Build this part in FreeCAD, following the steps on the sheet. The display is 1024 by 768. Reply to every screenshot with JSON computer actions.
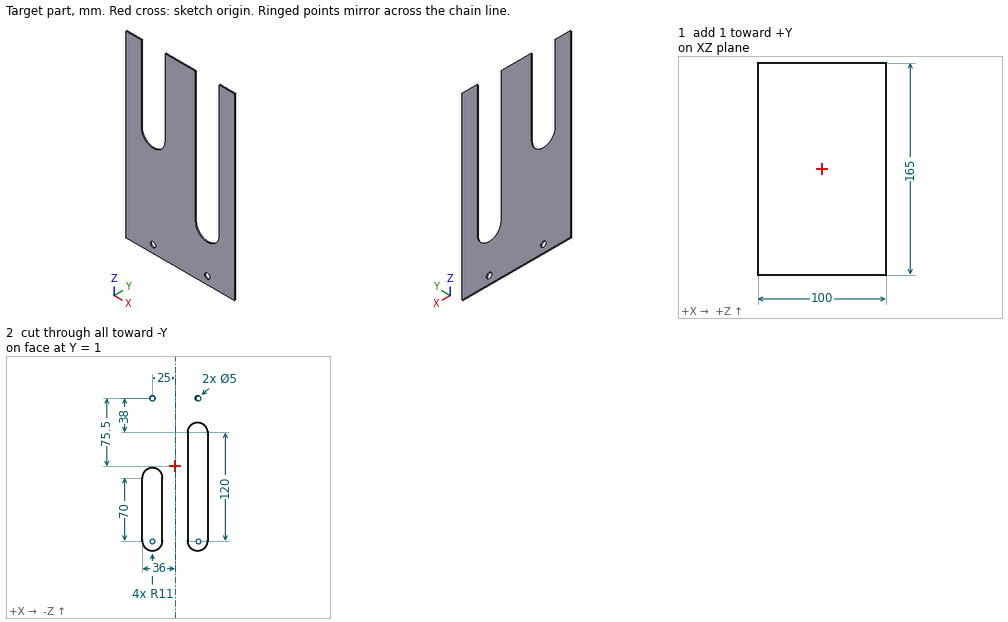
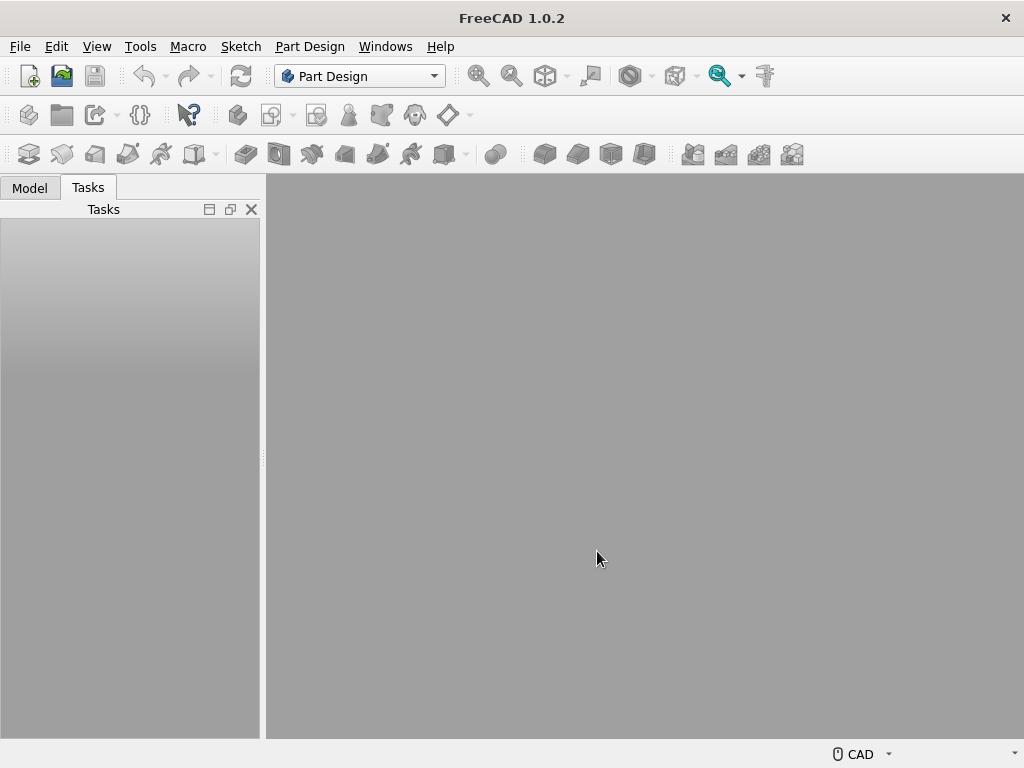
{"action": "left_click", "coordinate": [29, 76]}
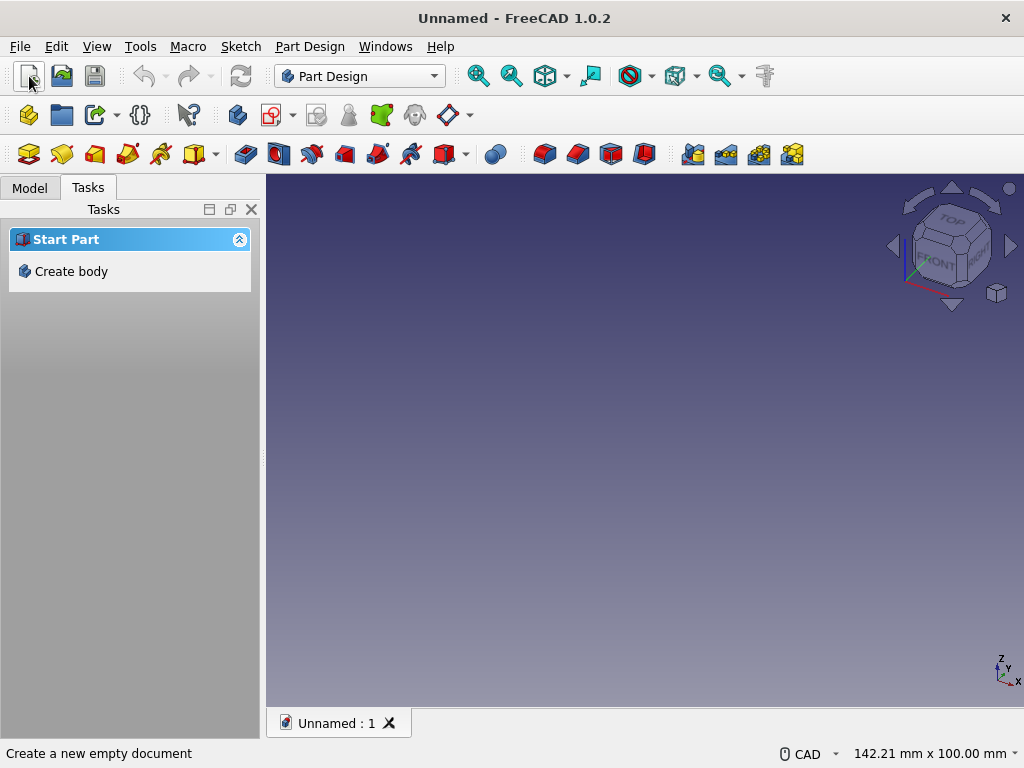
{"action": "left_click", "coordinate": [270, 116]}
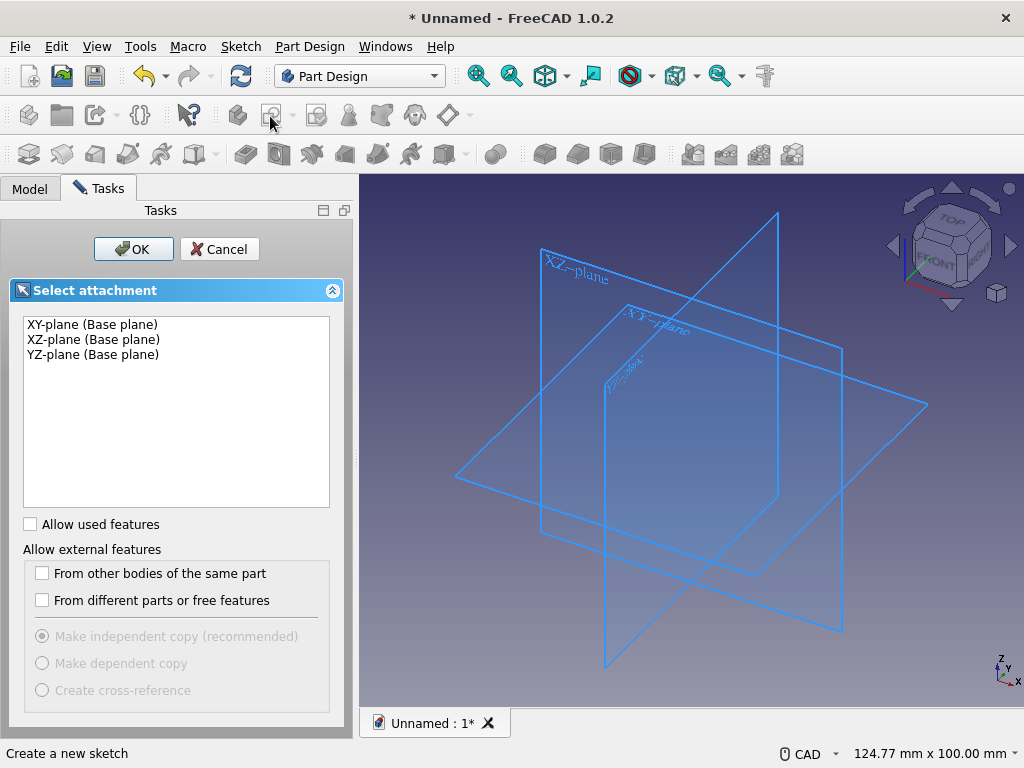
{"action": "left_click", "coordinate": [84, 340]}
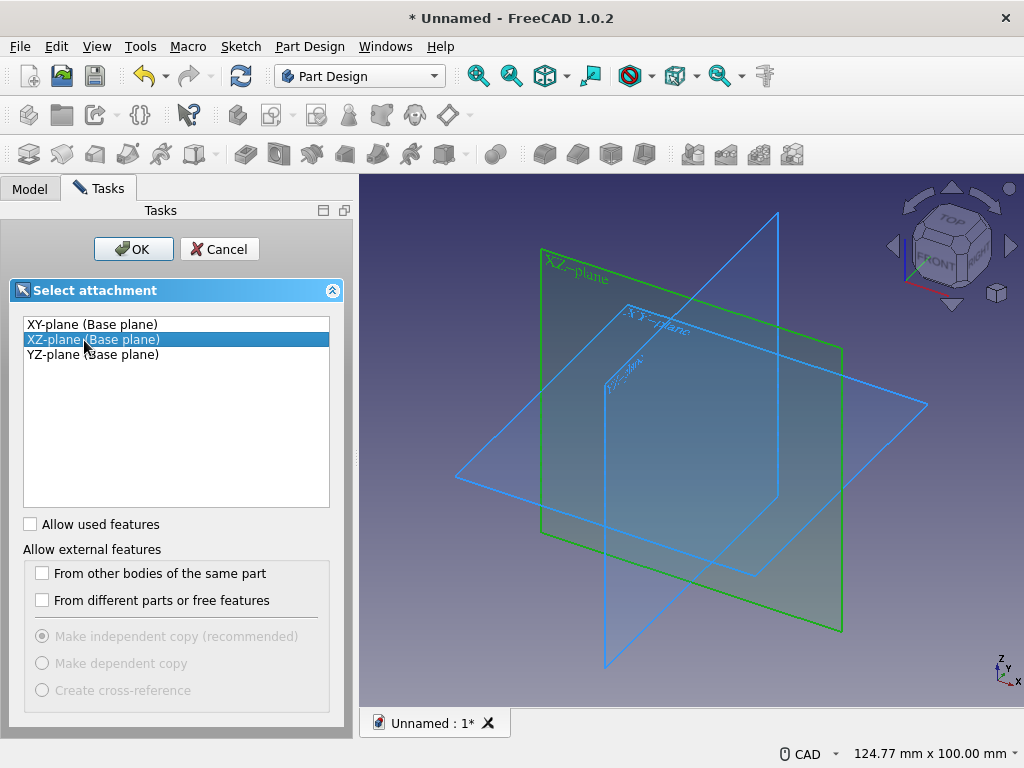
{"action": "left_click", "coordinate": [134, 249]}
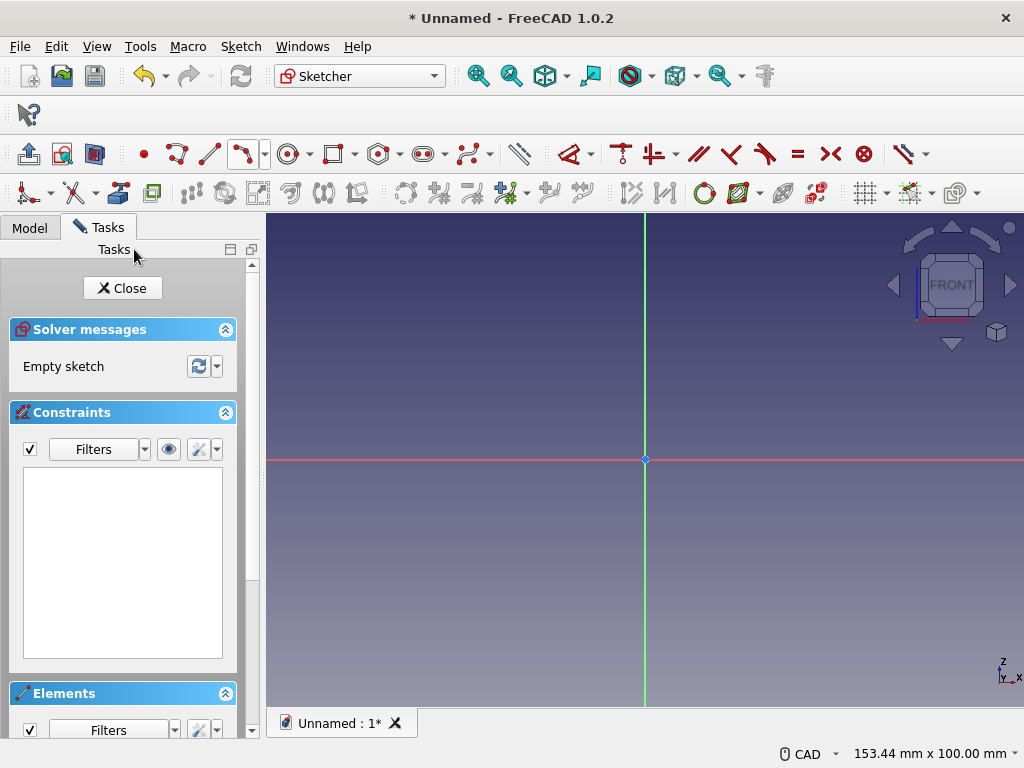
{"action": "scroll", "coordinate": [537, 460], "scroll_direction": "down", "scroll_amount": 5}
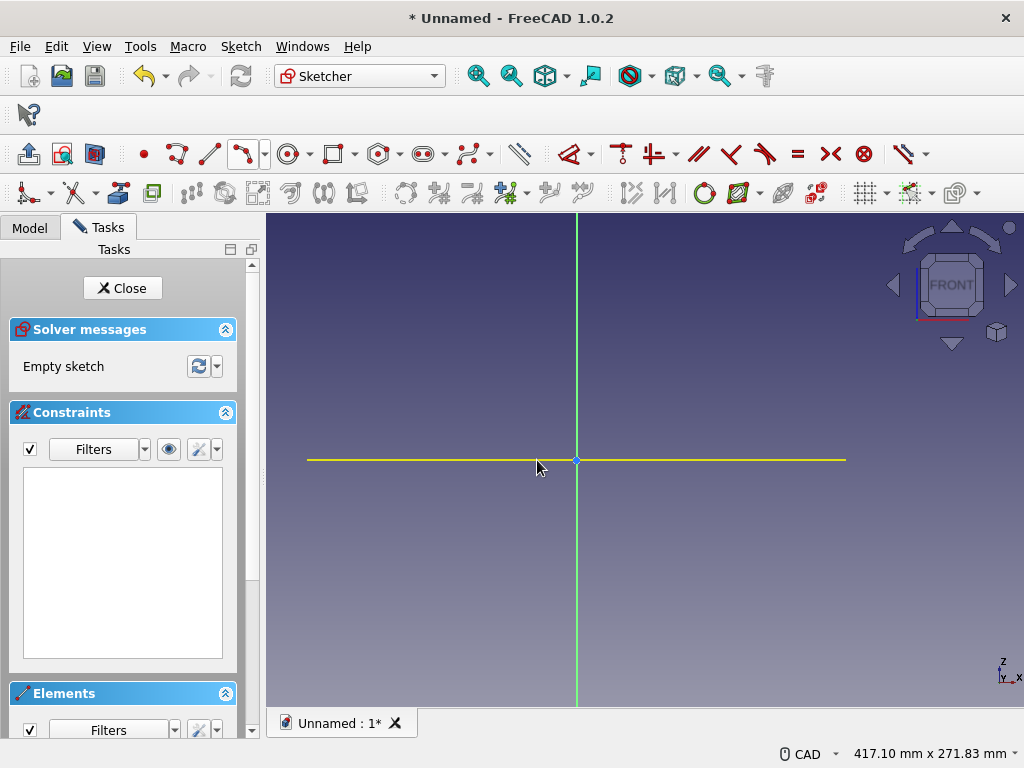
{"action": "left_click", "coordinate": [354, 154]}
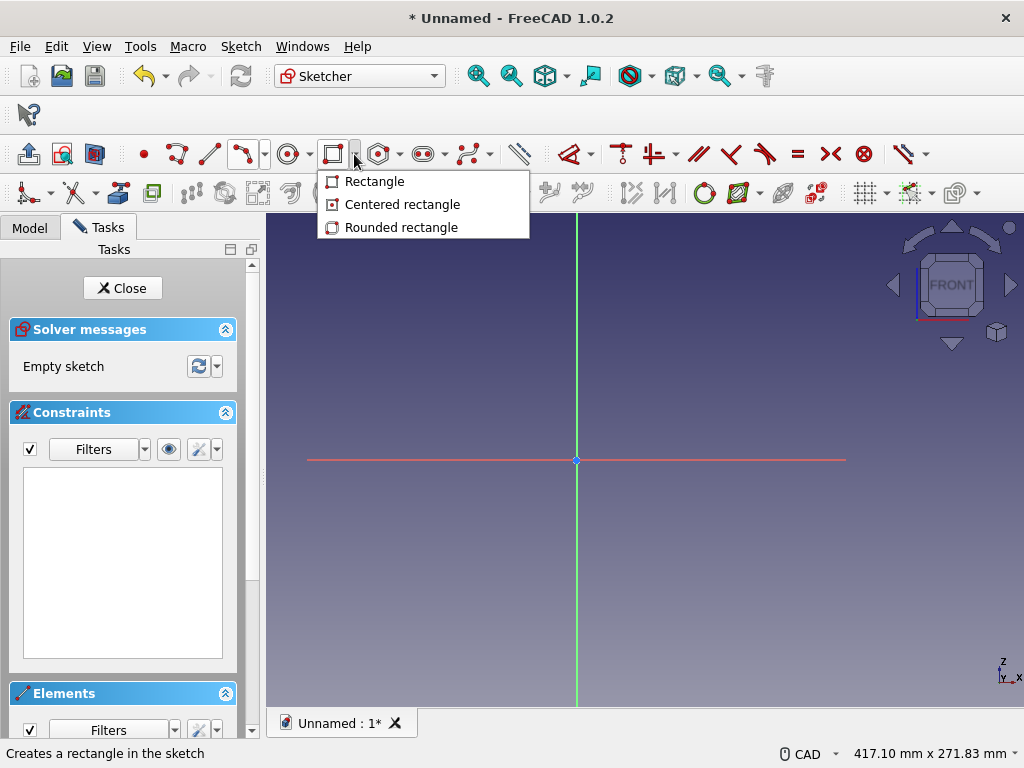
{"action": "left_click", "coordinate": [424, 204]}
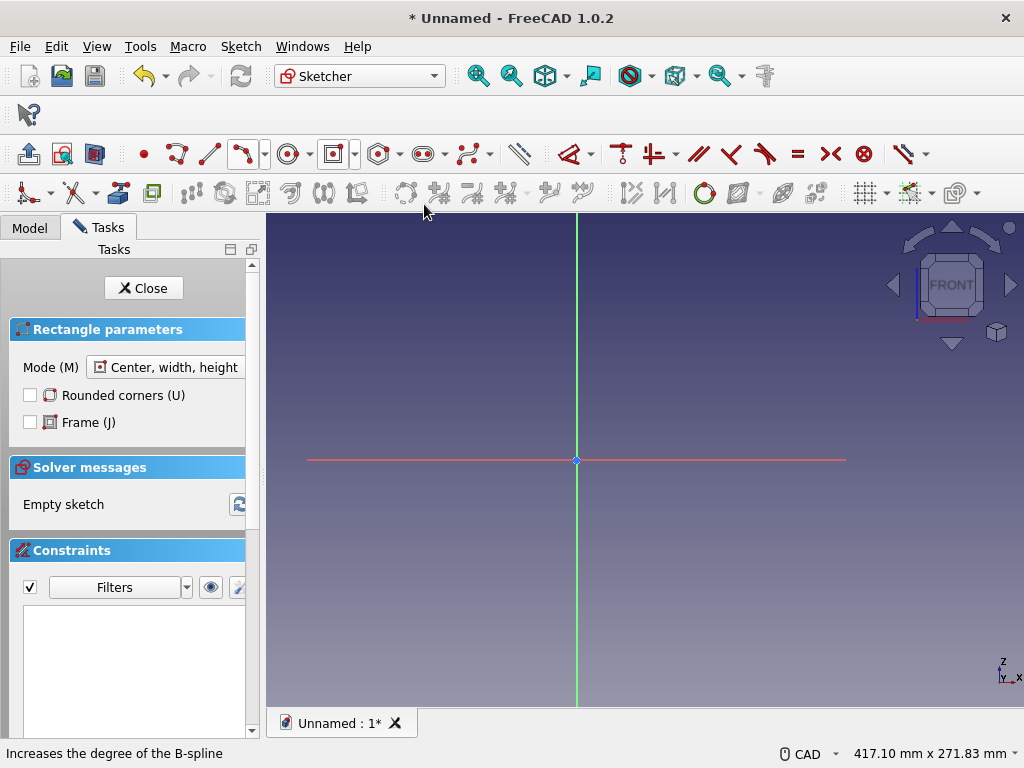
{"action": "left_click", "coordinate": [577, 460]}
{"action": "left_click", "coordinate": [668, 310]}
{"action": "key", "text": "Escape"}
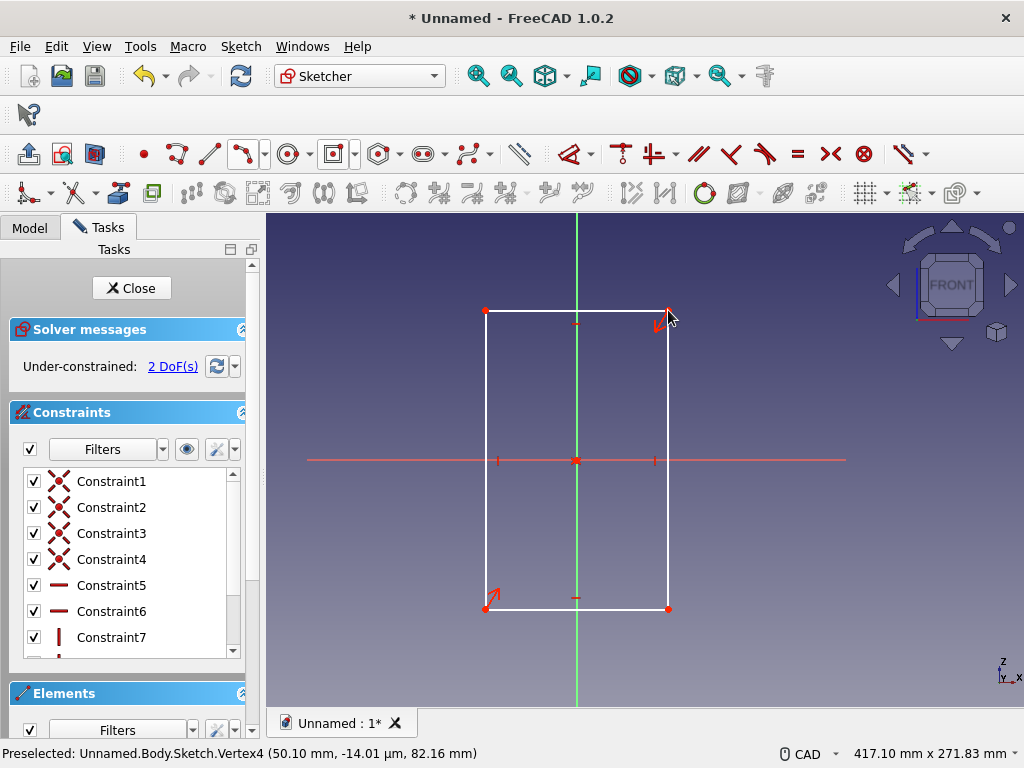
{"action": "left_click", "coordinate": [541, 610]}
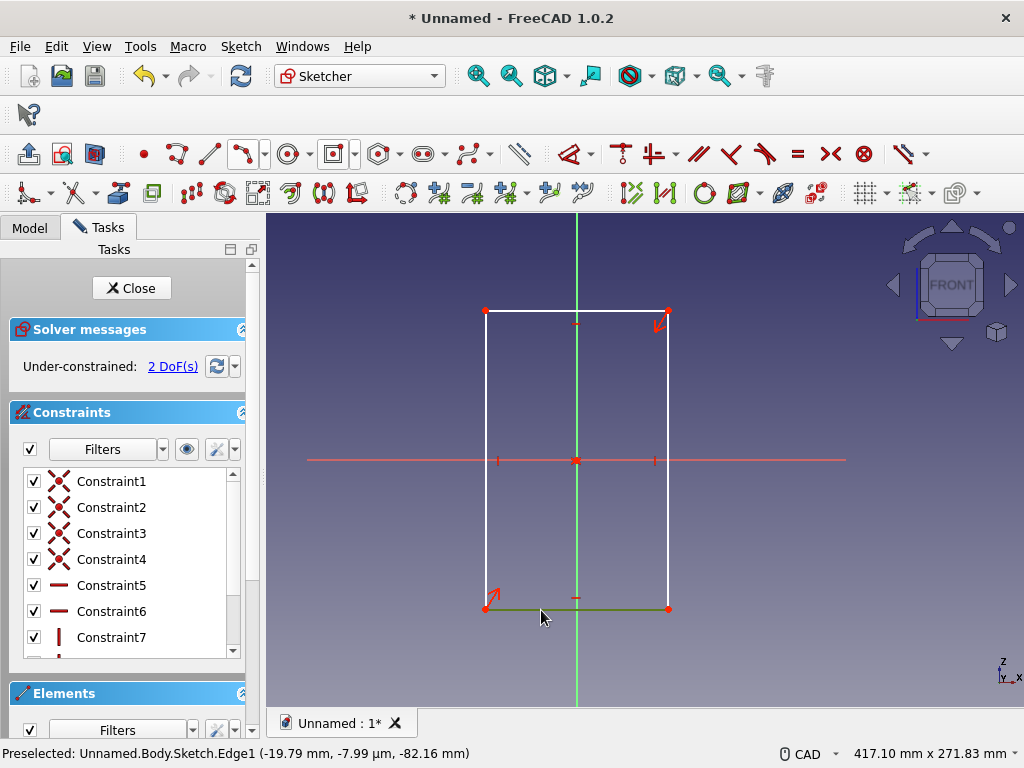
{"action": "key", "text": "l"}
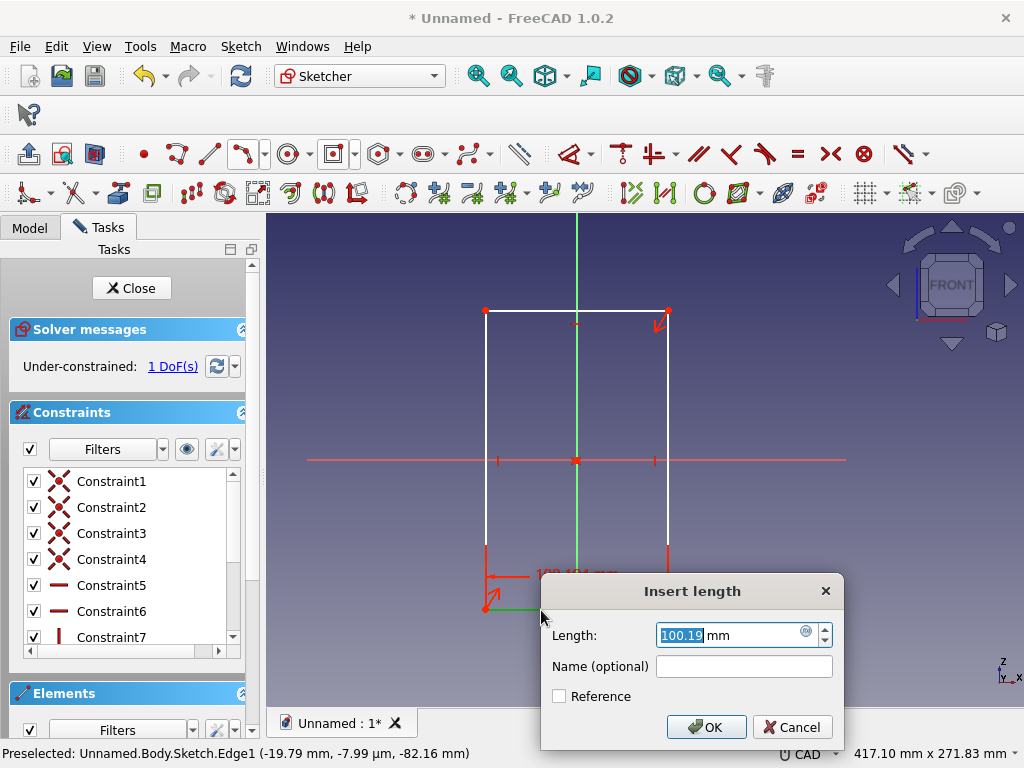
{"action": "type", "text": "100"}
{"action": "key", "text": "Return"}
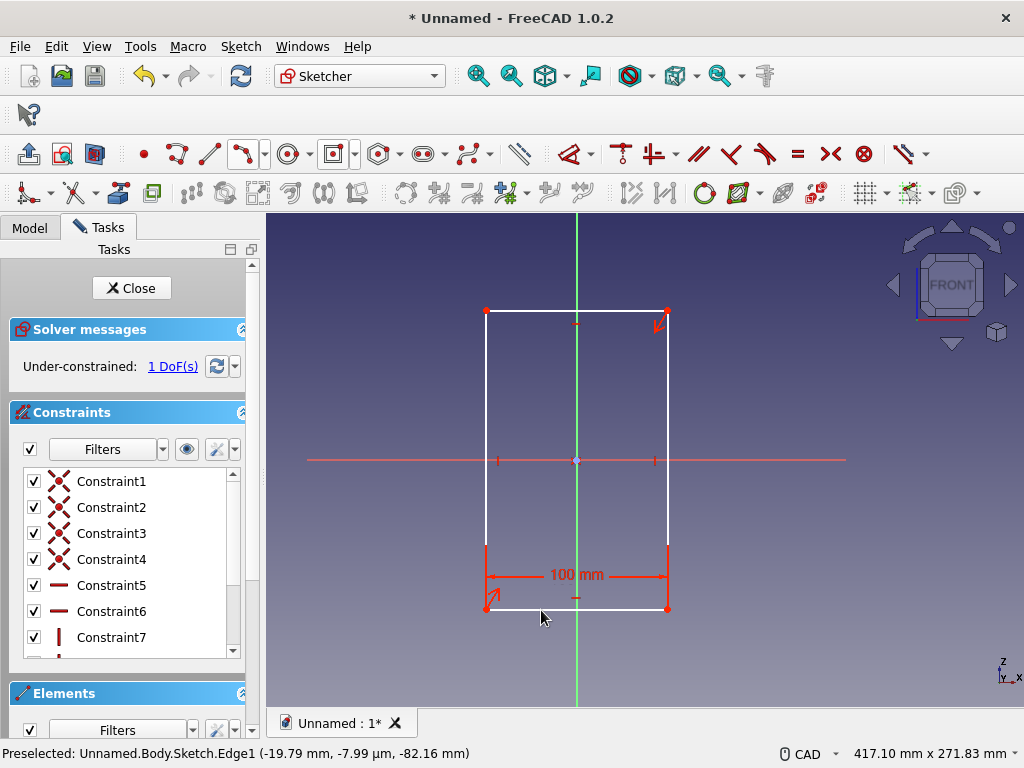
{"action": "left_click", "coordinate": [668, 520]}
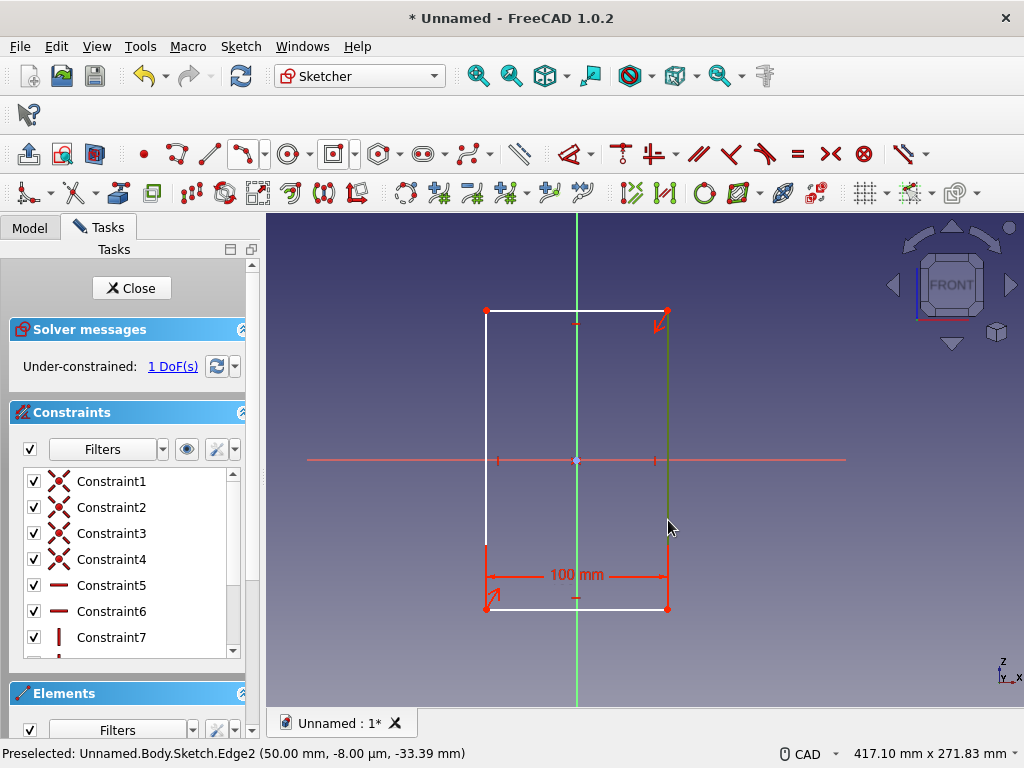
{"action": "left_click", "coordinate": [590, 154]}